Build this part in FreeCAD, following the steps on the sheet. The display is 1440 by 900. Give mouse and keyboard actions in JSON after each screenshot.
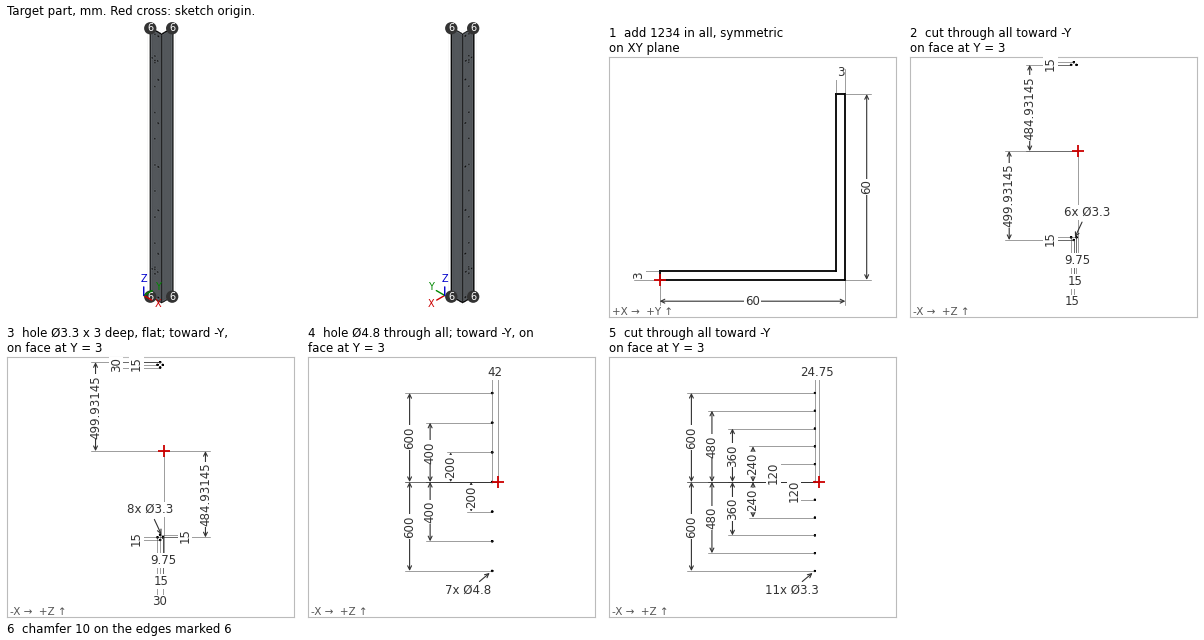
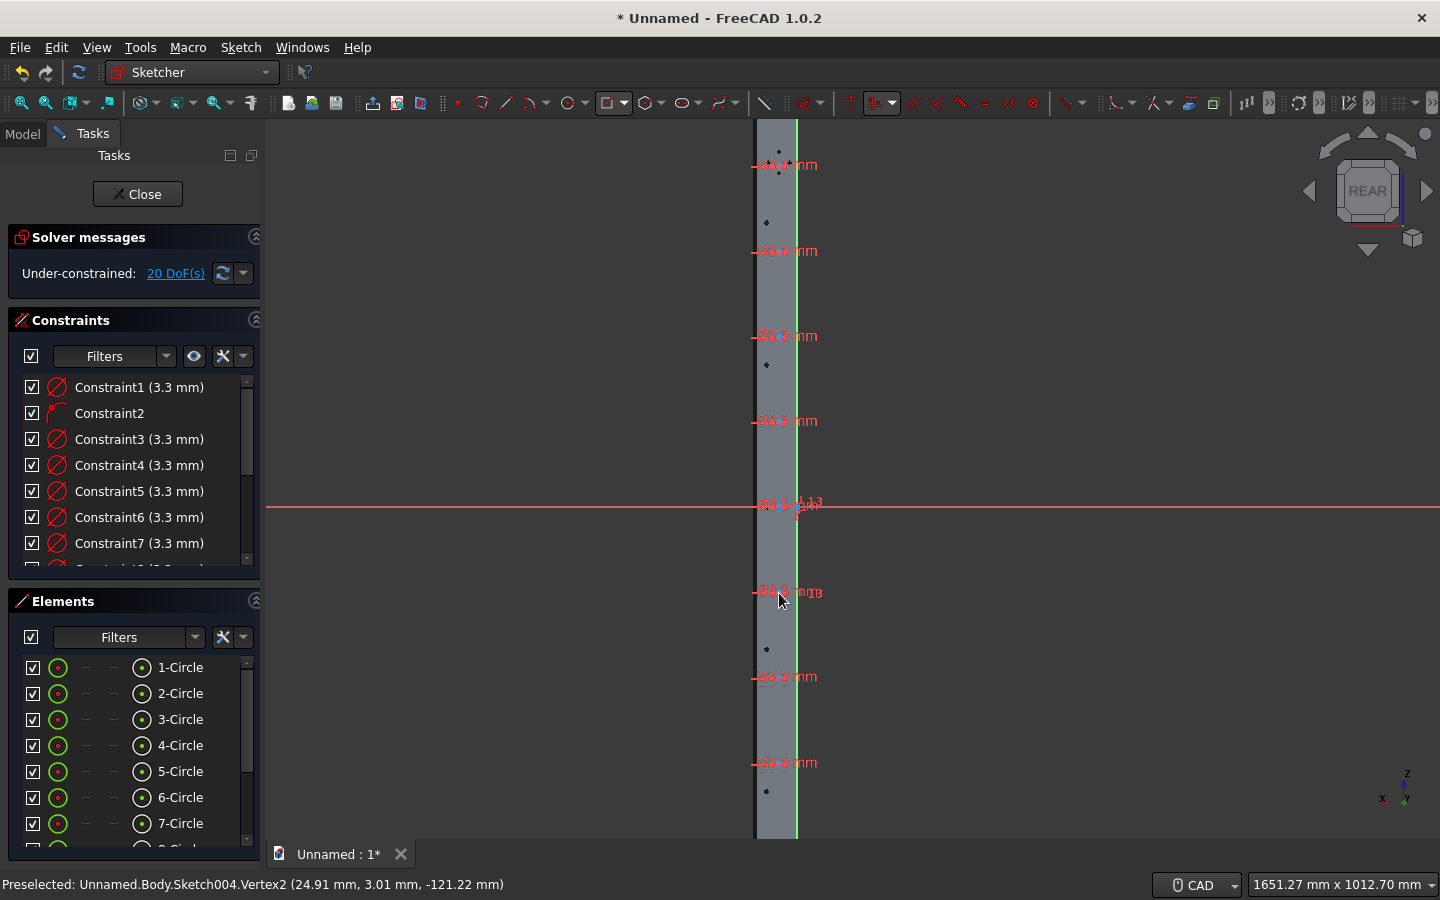
{"action": "left_click", "coordinate": [779, 593]}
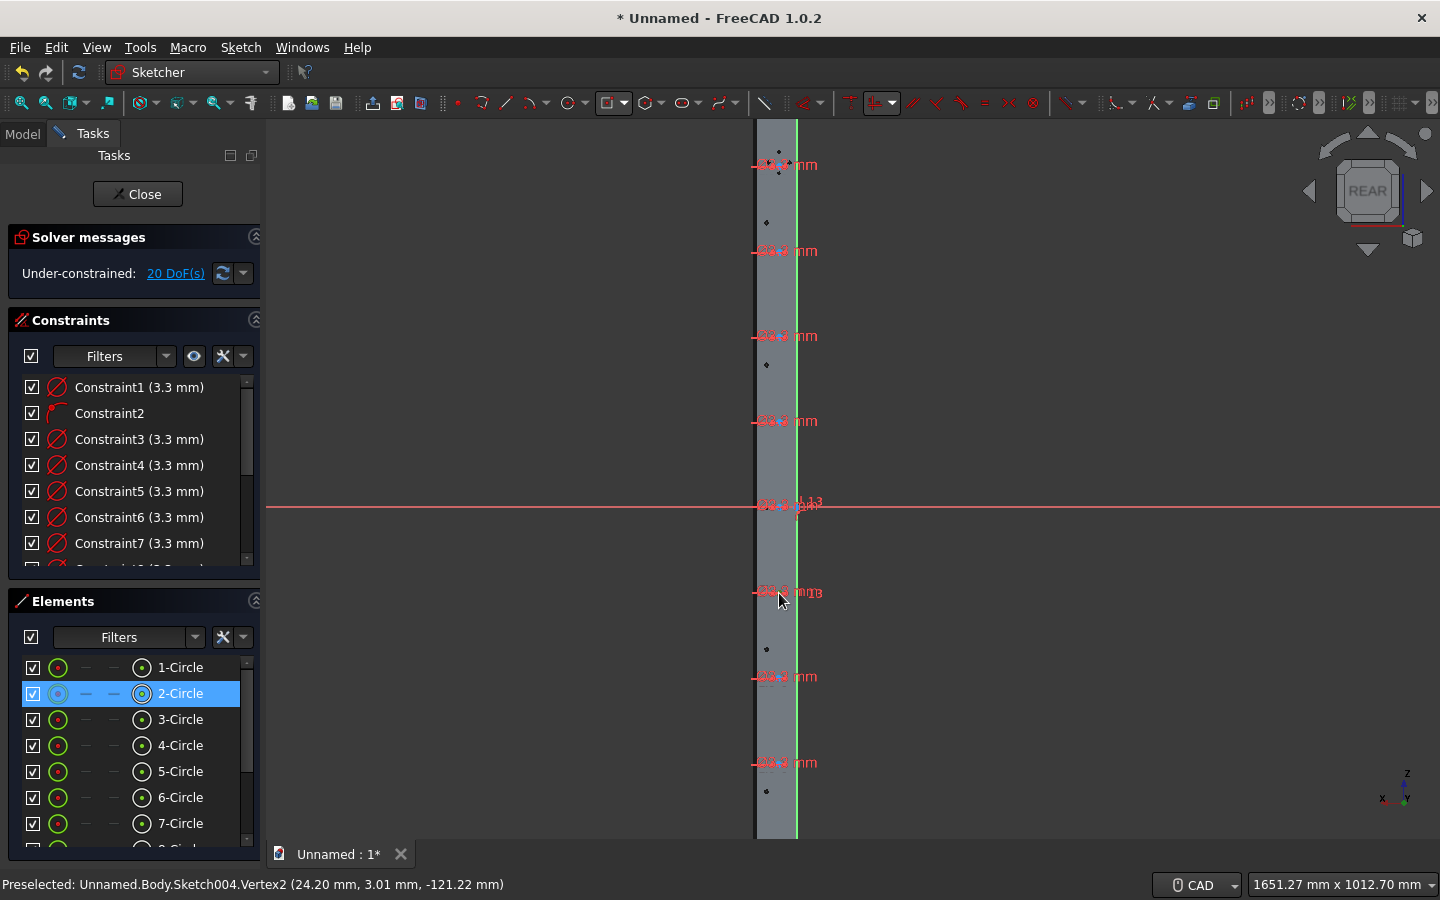
{"action": "left_click", "coordinate": [779, 679]}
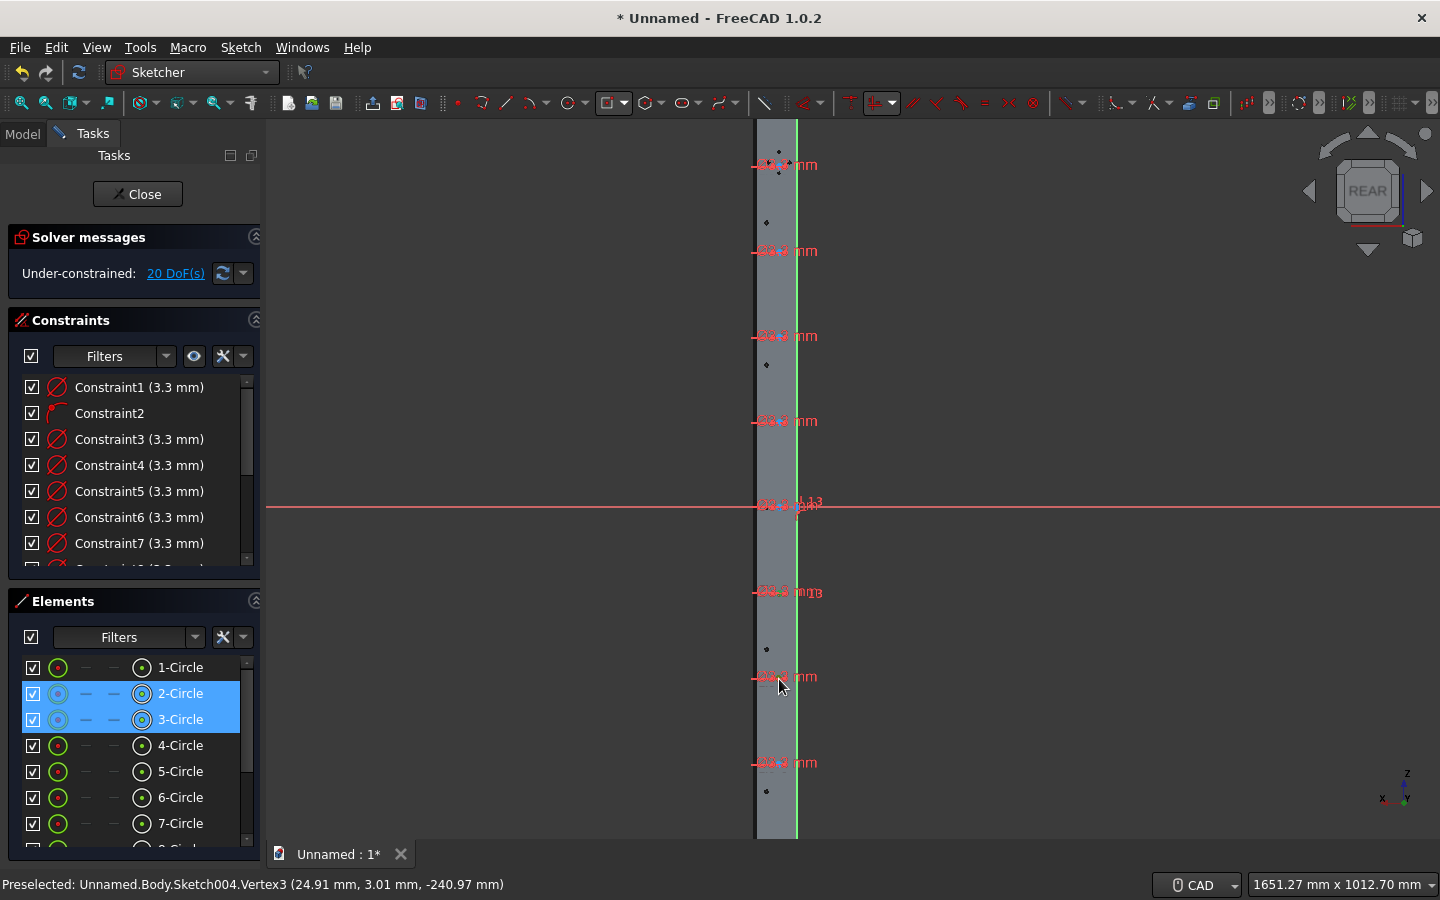
{"action": "key", "text": "v"}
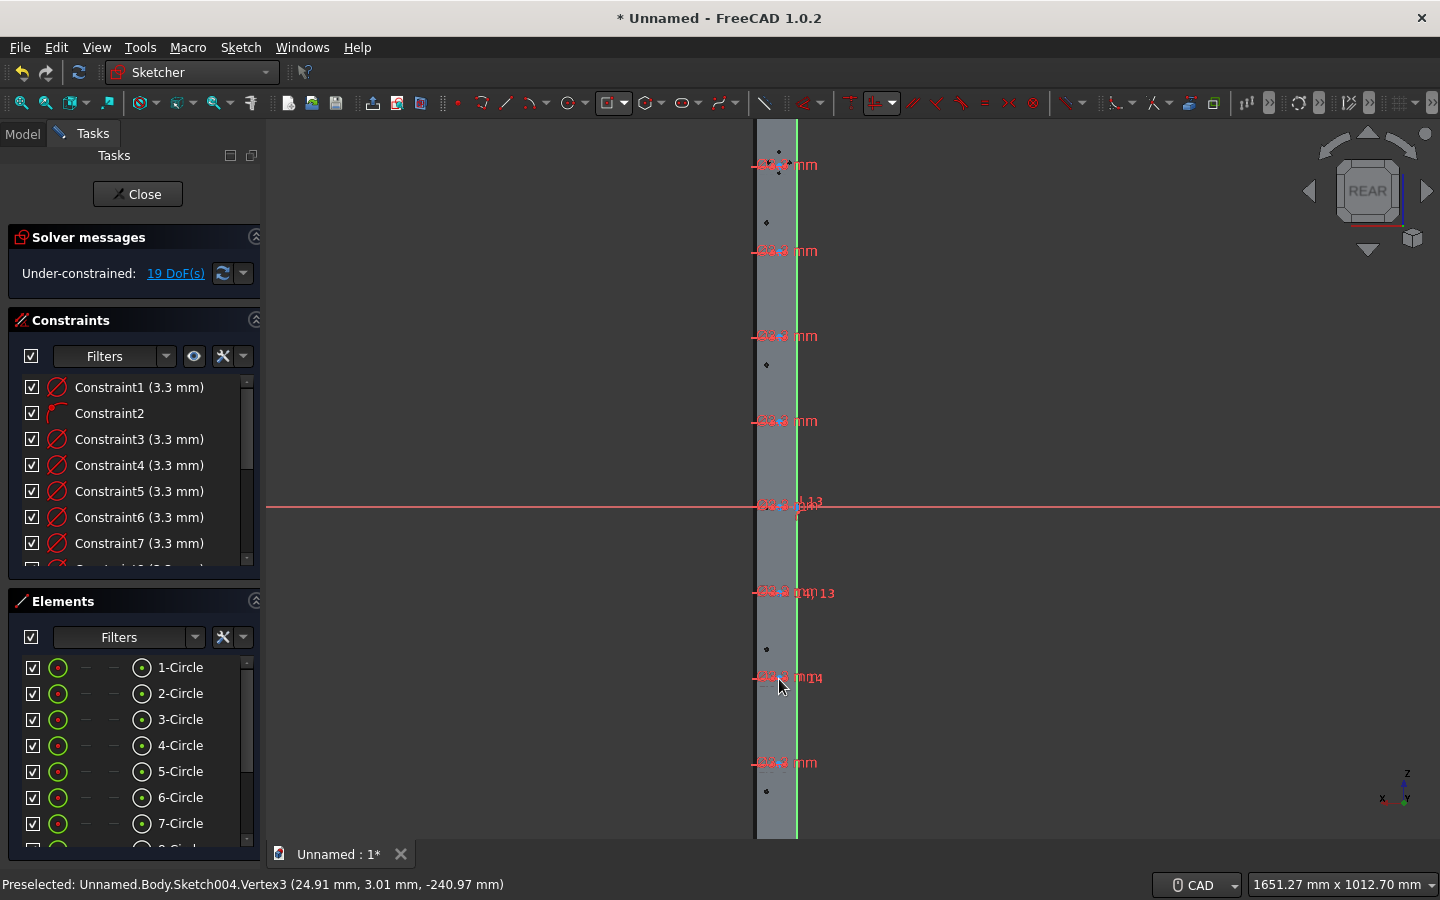
{"action": "left_click", "coordinate": [779, 679]}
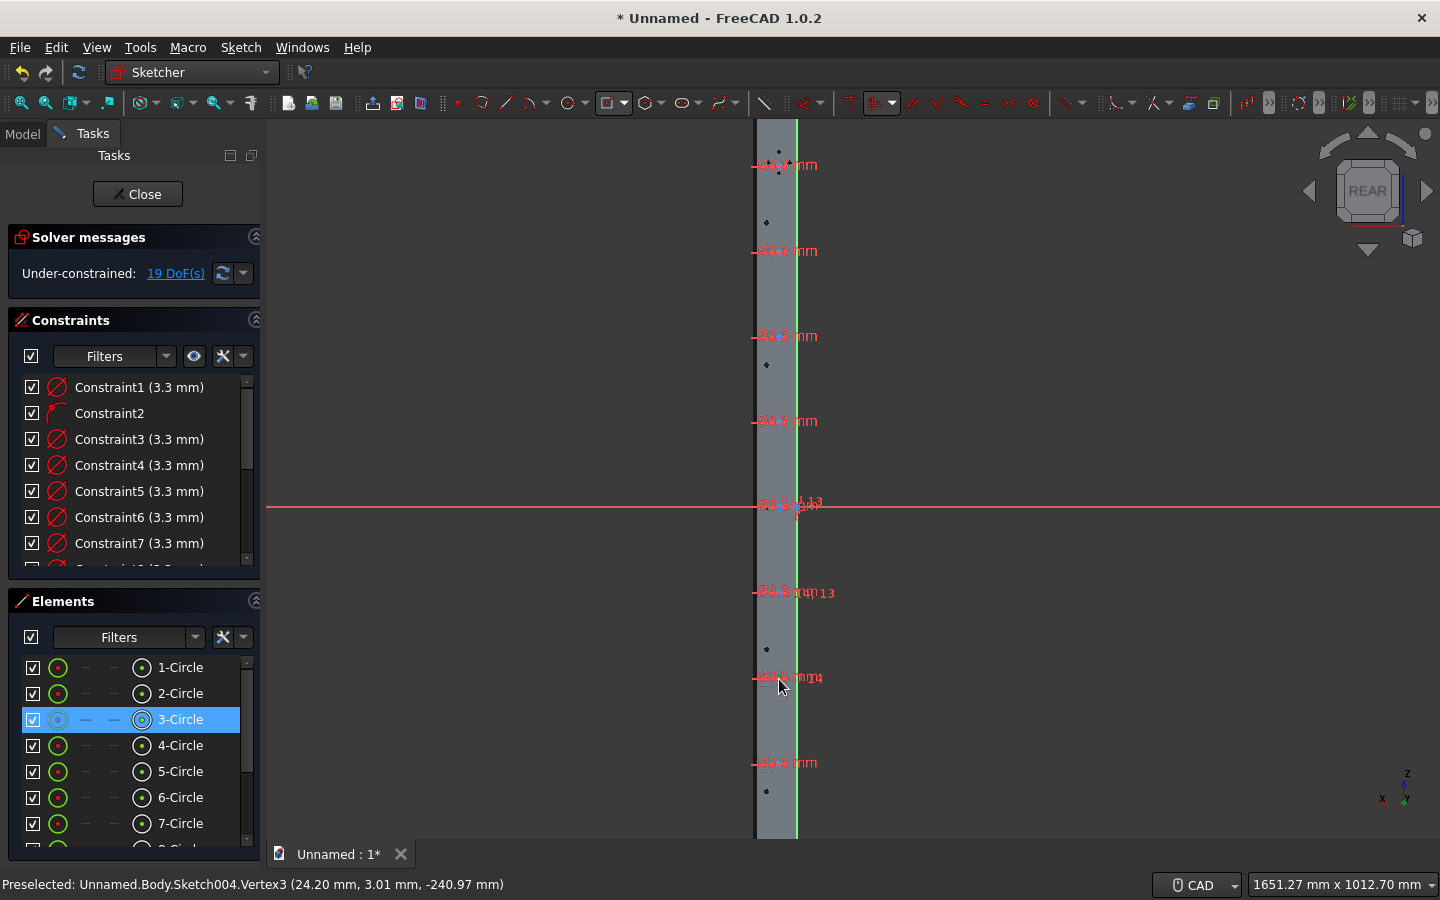
{"action": "left_click", "coordinate": [779, 765]}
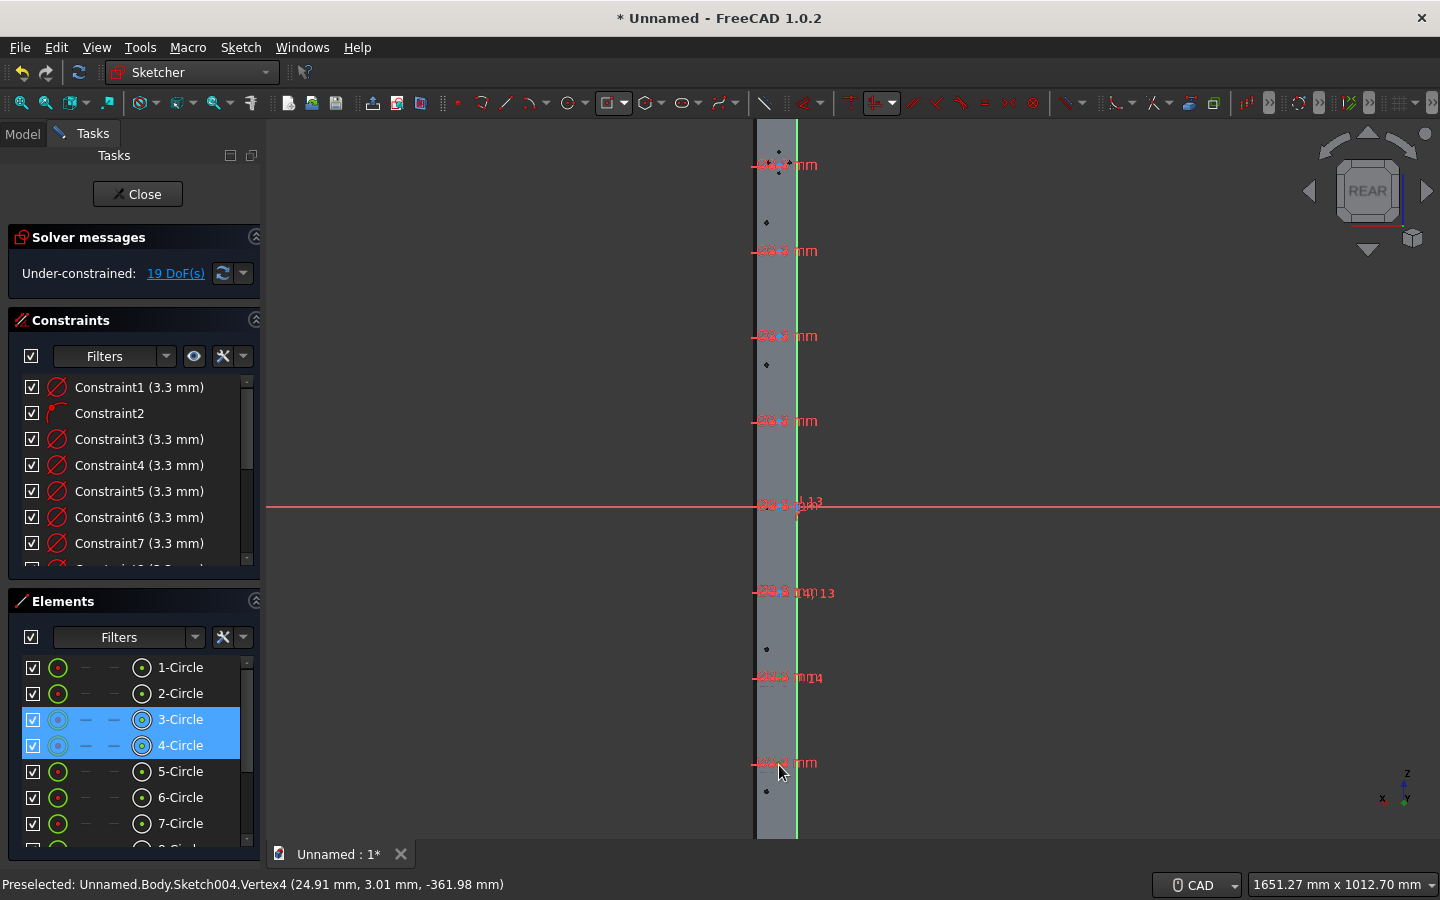
{"action": "left_click", "coordinate": [894, 104]}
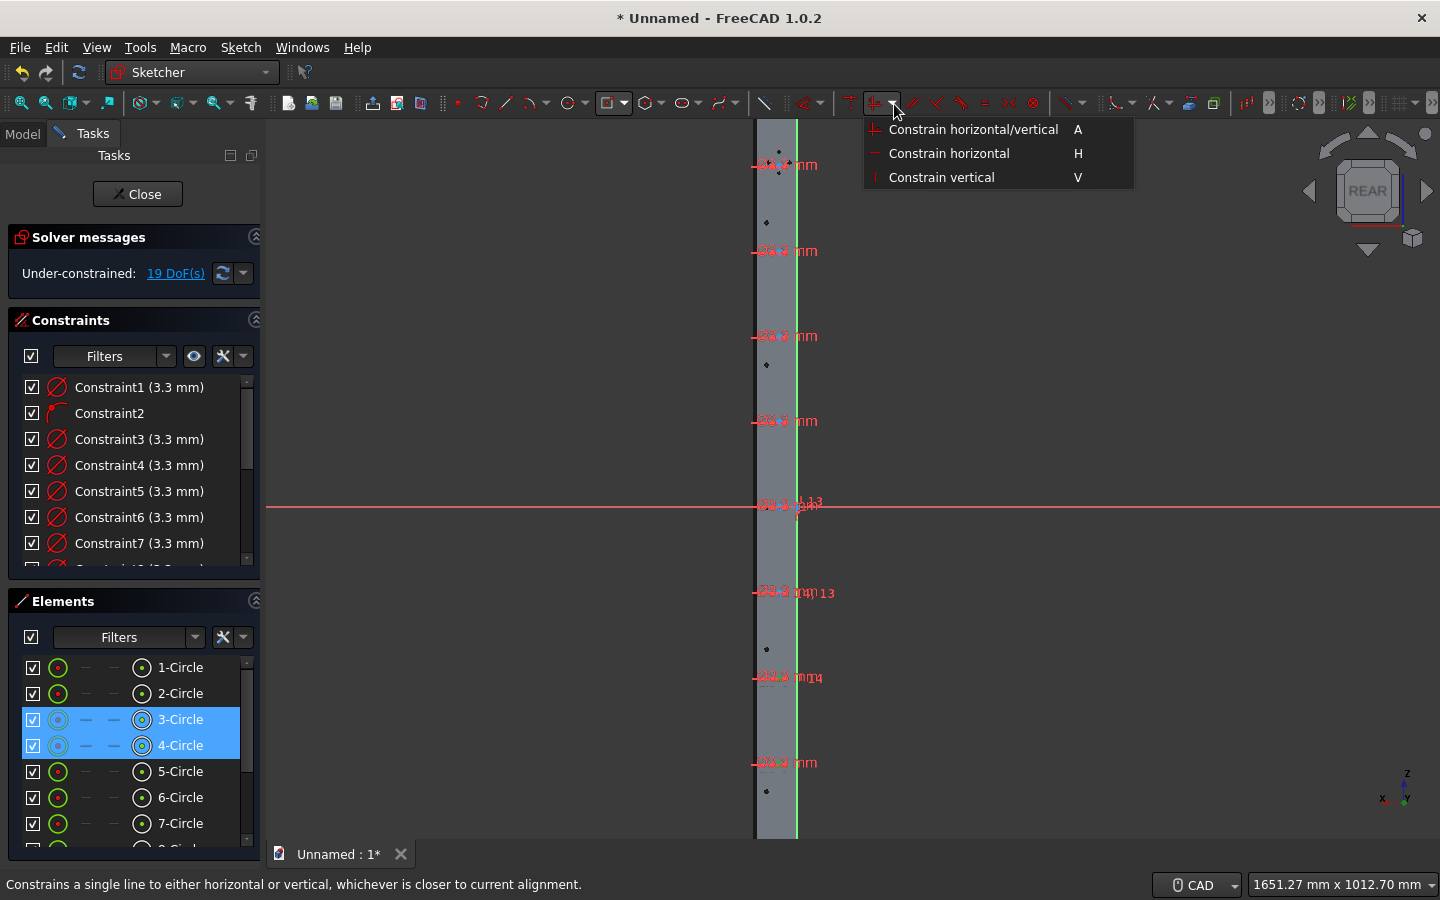
{"action": "left_click", "coordinate": [999, 177]}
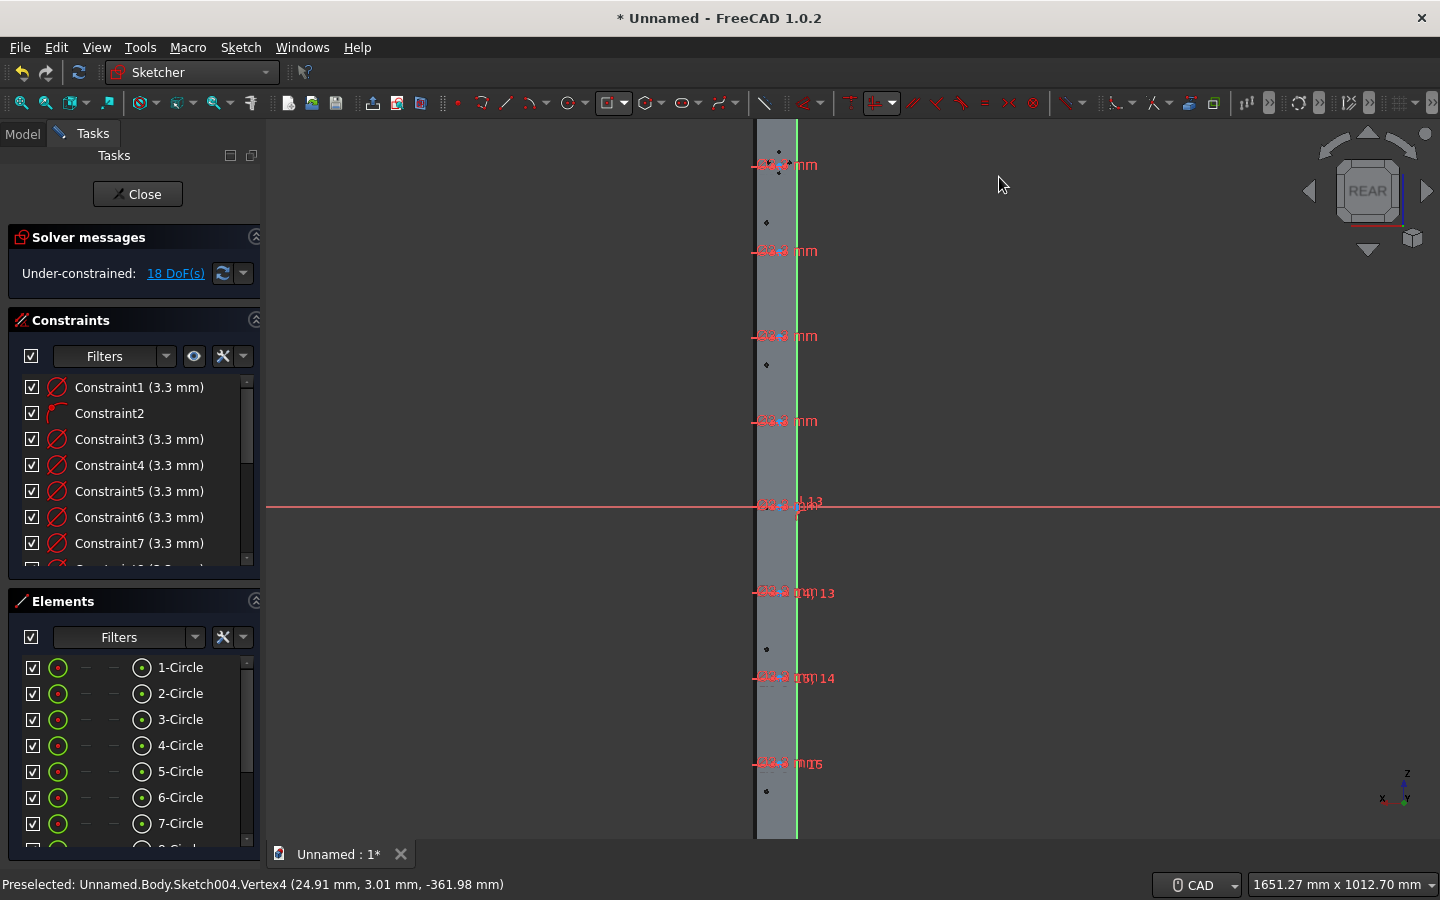
{"action": "left_click", "coordinate": [779, 765]}